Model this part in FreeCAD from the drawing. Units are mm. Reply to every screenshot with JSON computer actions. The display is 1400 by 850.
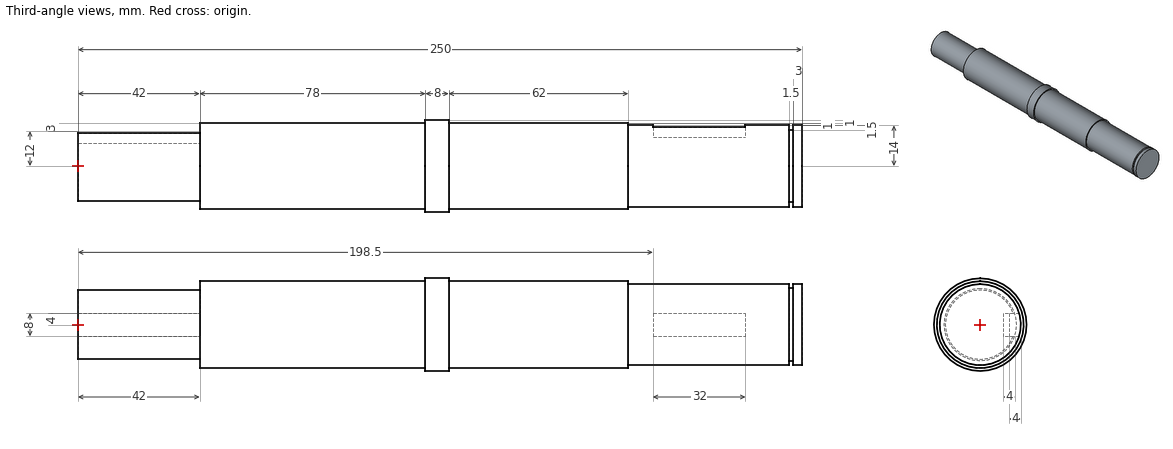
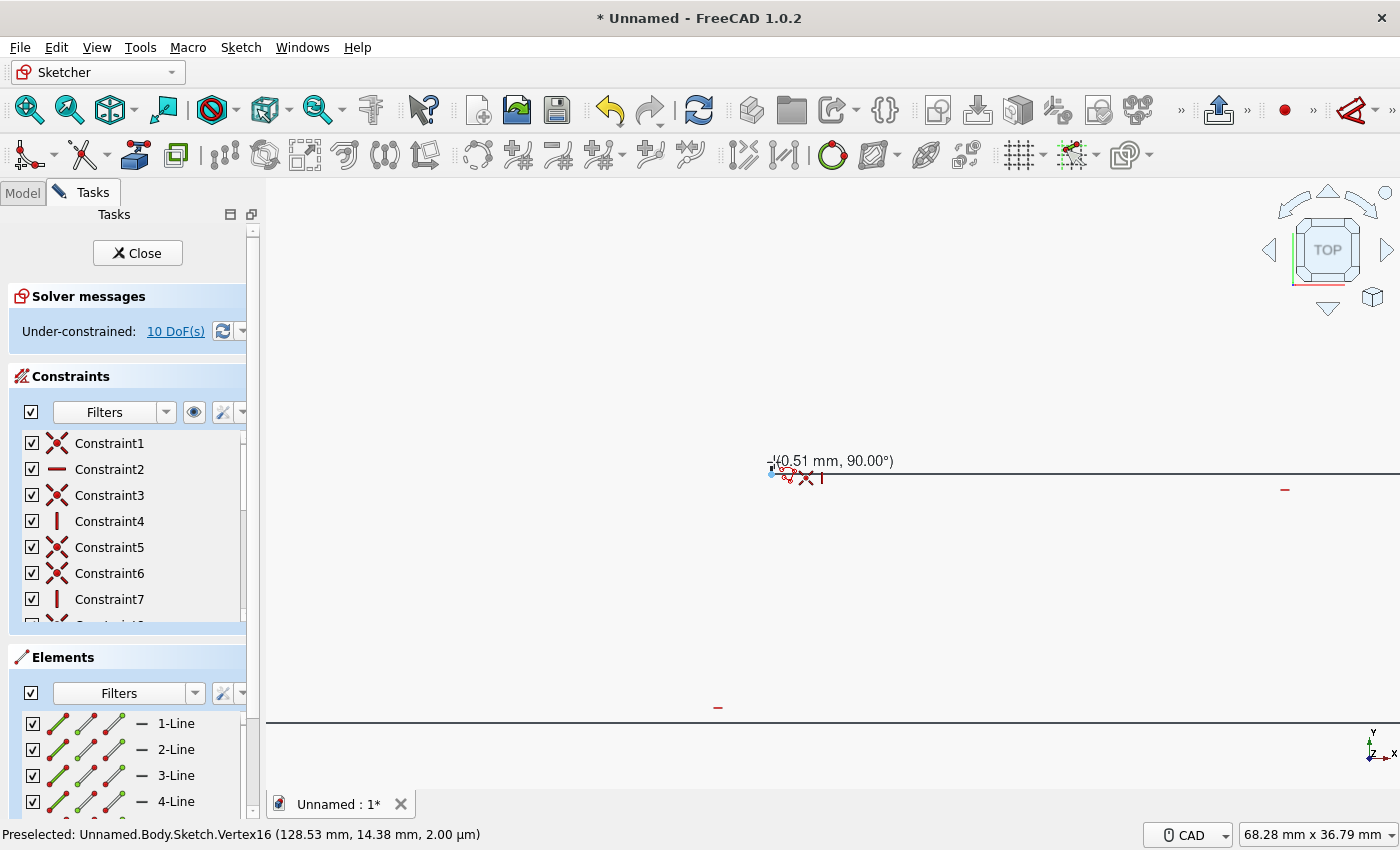
{"action": "left_click", "coordinate": [772, 457]}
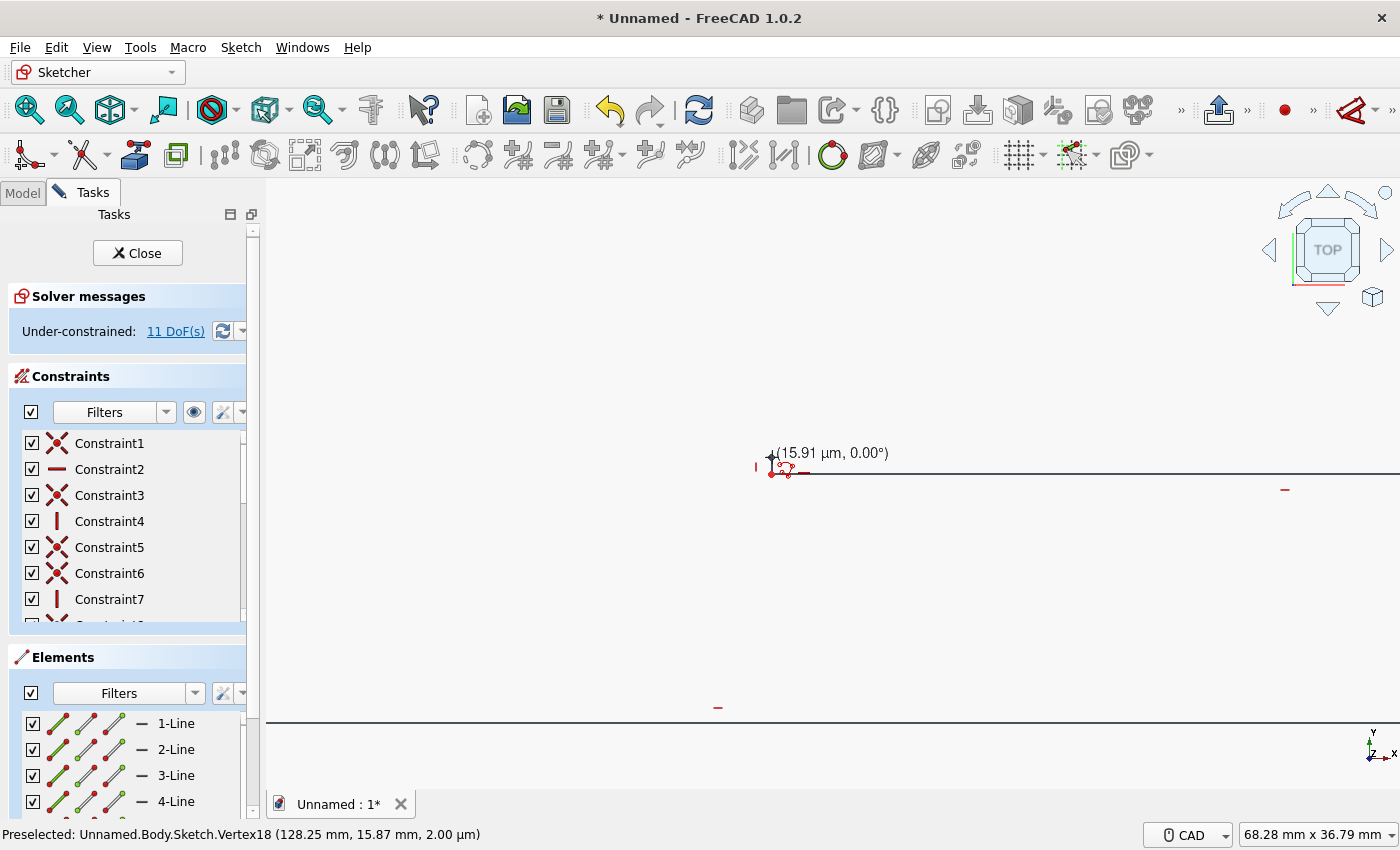
{"action": "scroll", "coordinate": [773, 462], "scroll_direction": "down", "scroll_amount": 9}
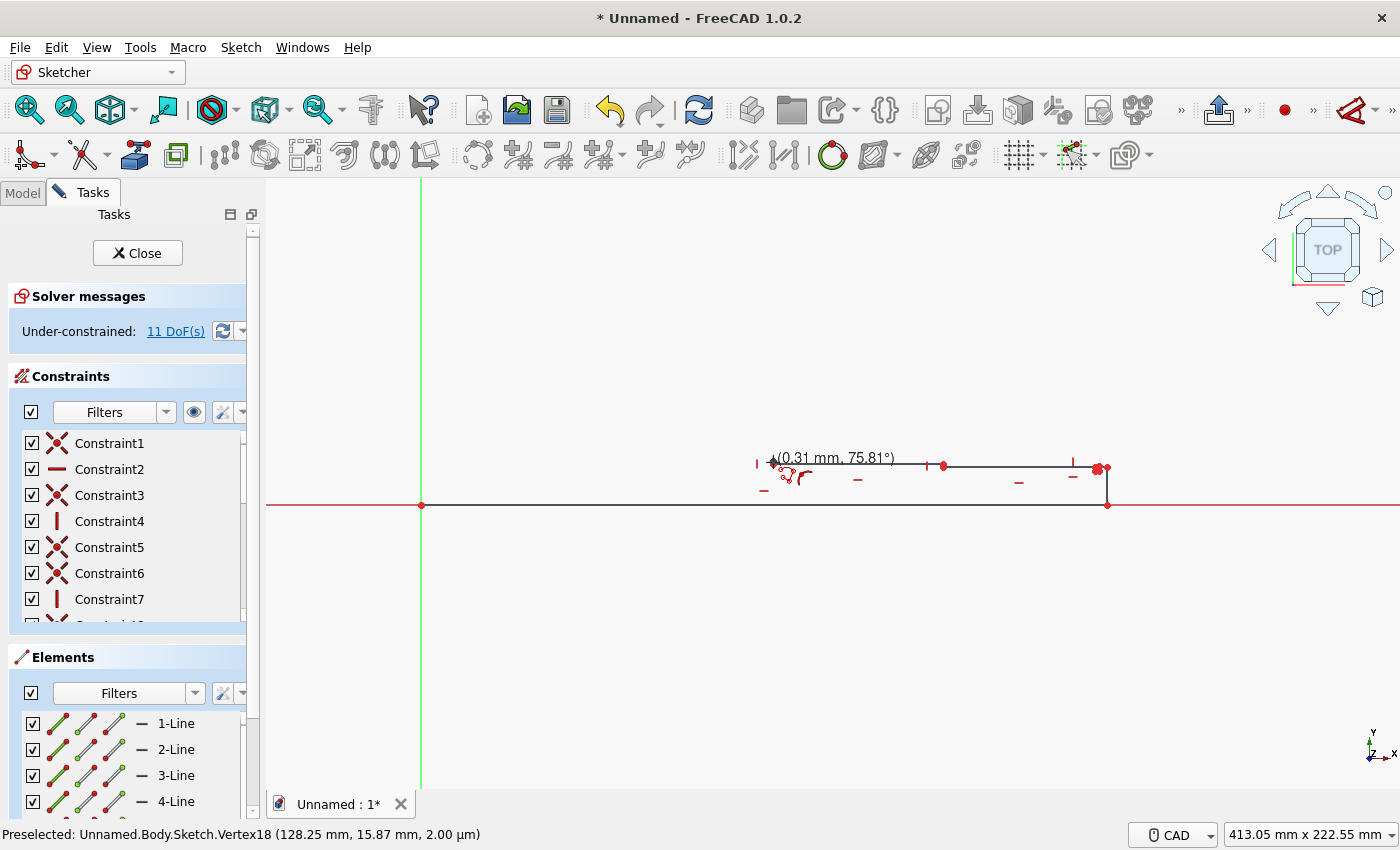
{"action": "left_click", "coordinate": [751, 462]}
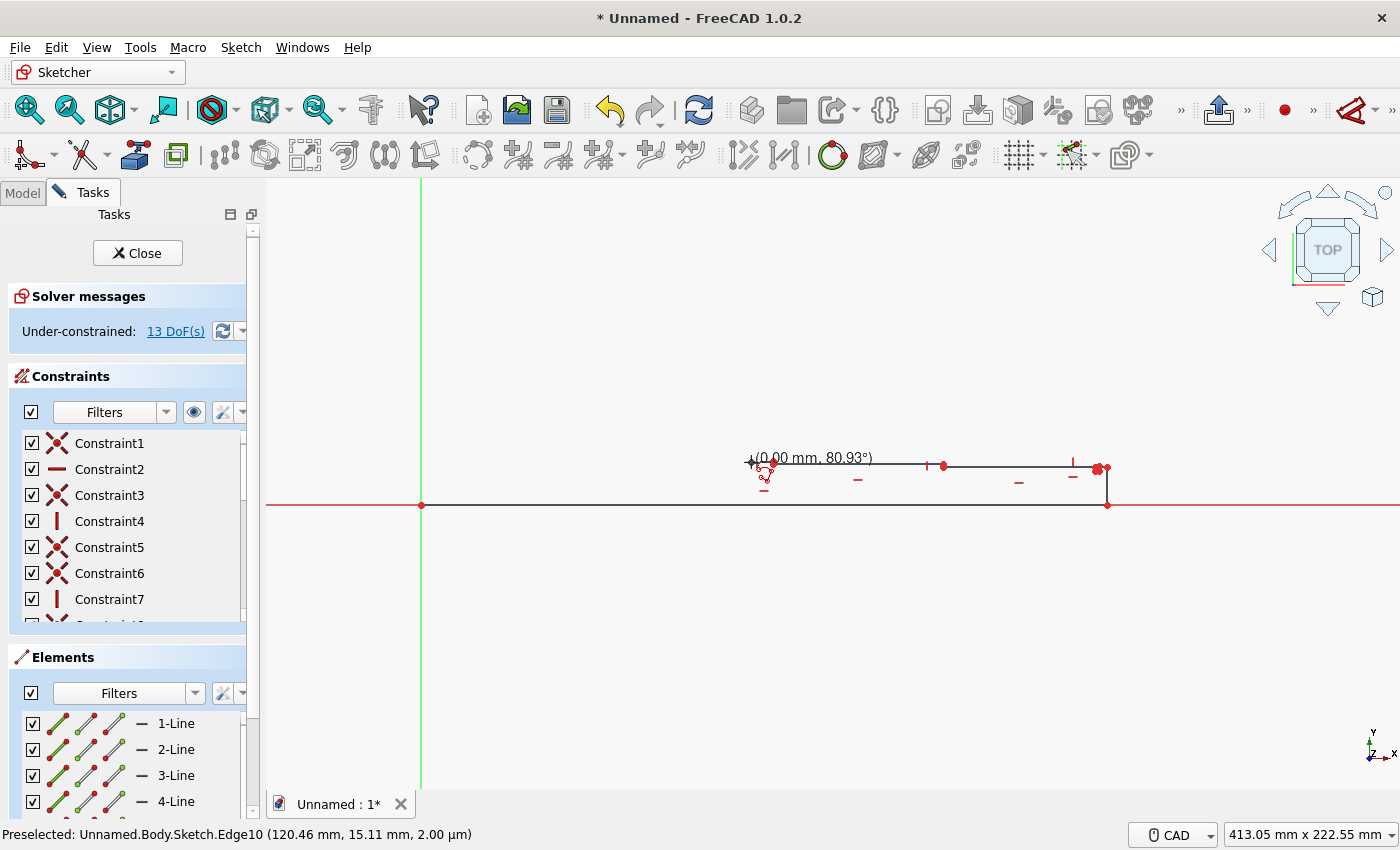
{"action": "scroll", "coordinate": [751, 464], "scroll_direction": "up", "scroll_amount": 9}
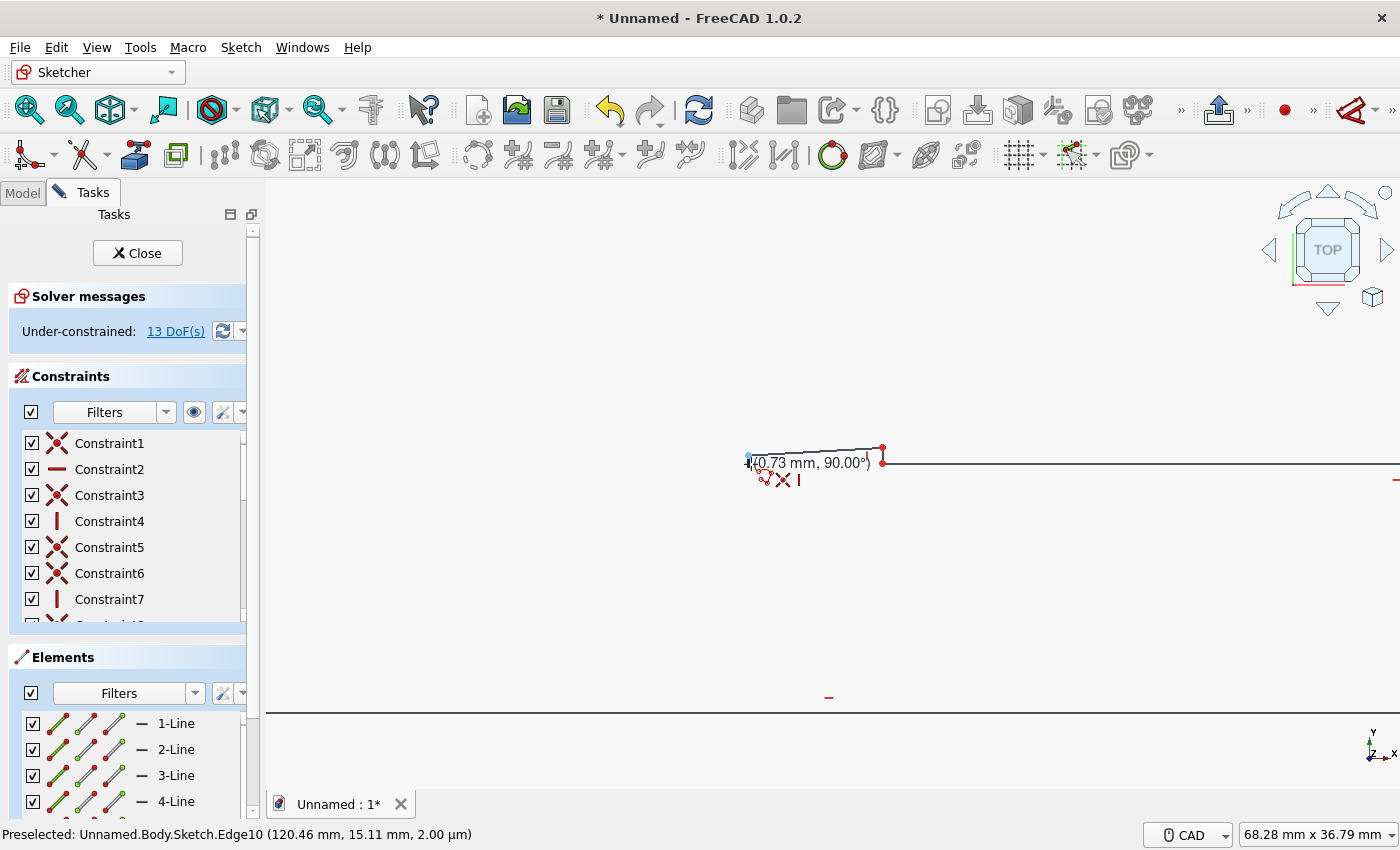
{"action": "left_click", "coordinate": [749, 463]}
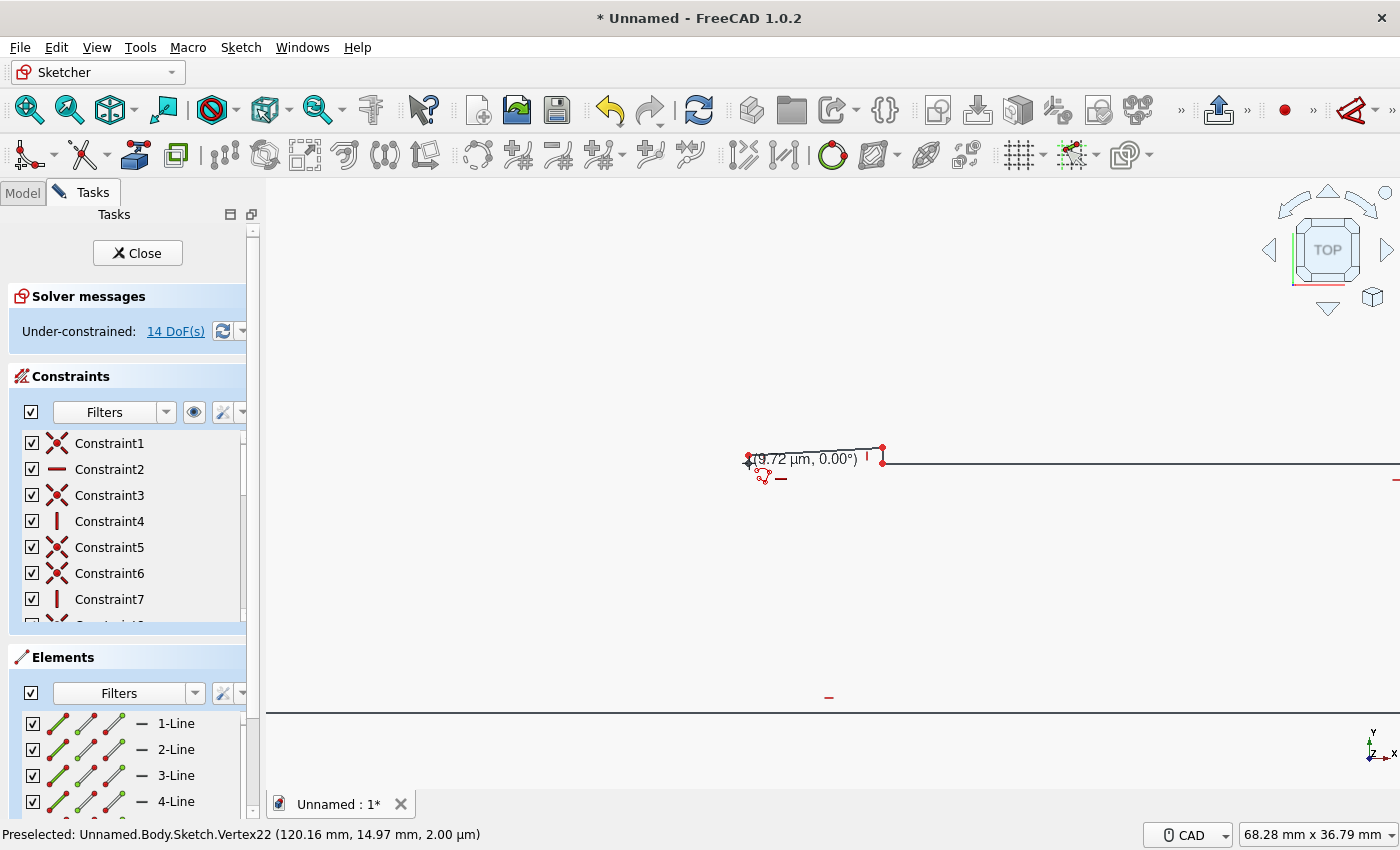
{"action": "scroll", "coordinate": [751, 464], "scroll_direction": "down", "scroll_amount": 9}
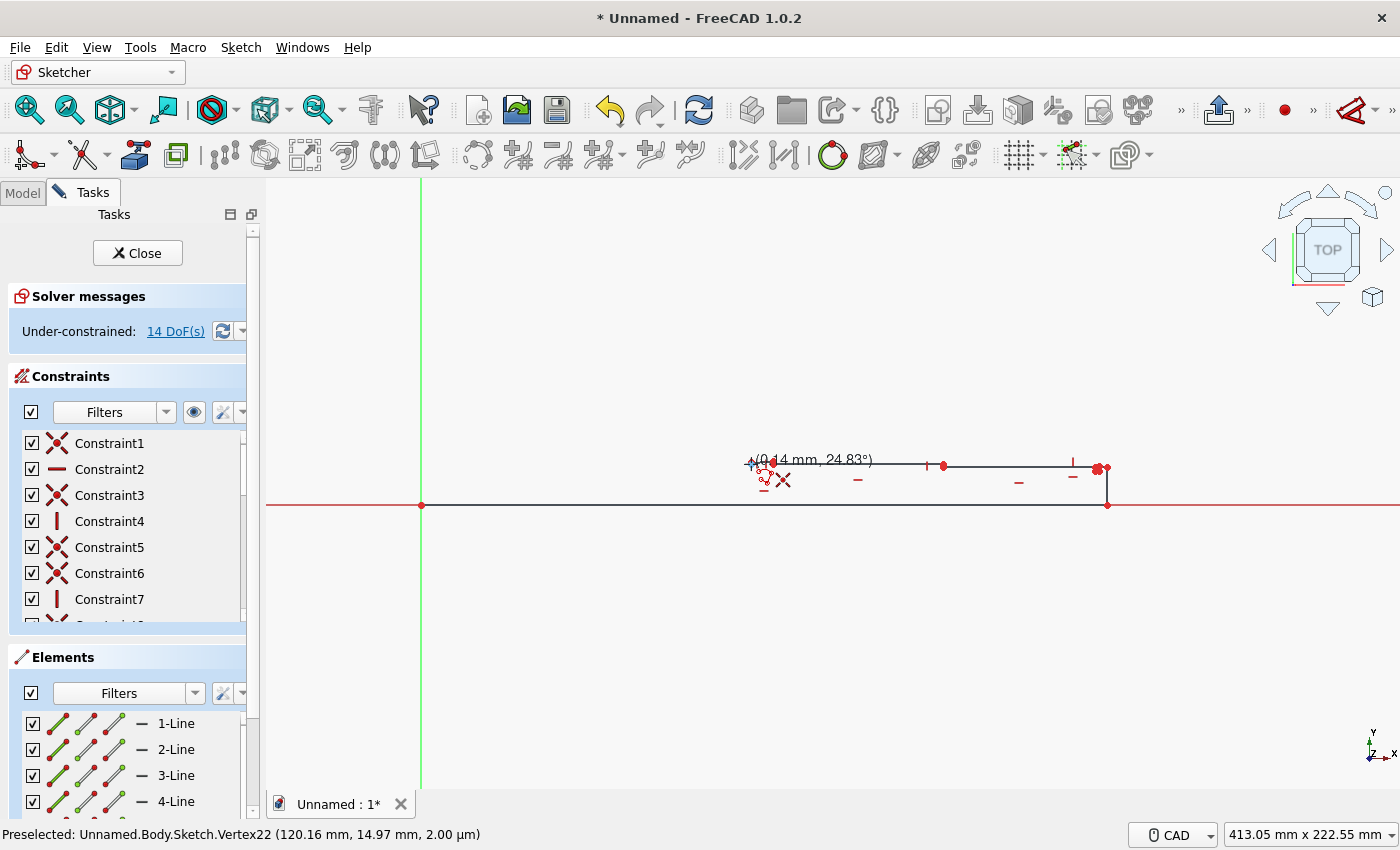
{"action": "left_click", "coordinate": [537, 464]}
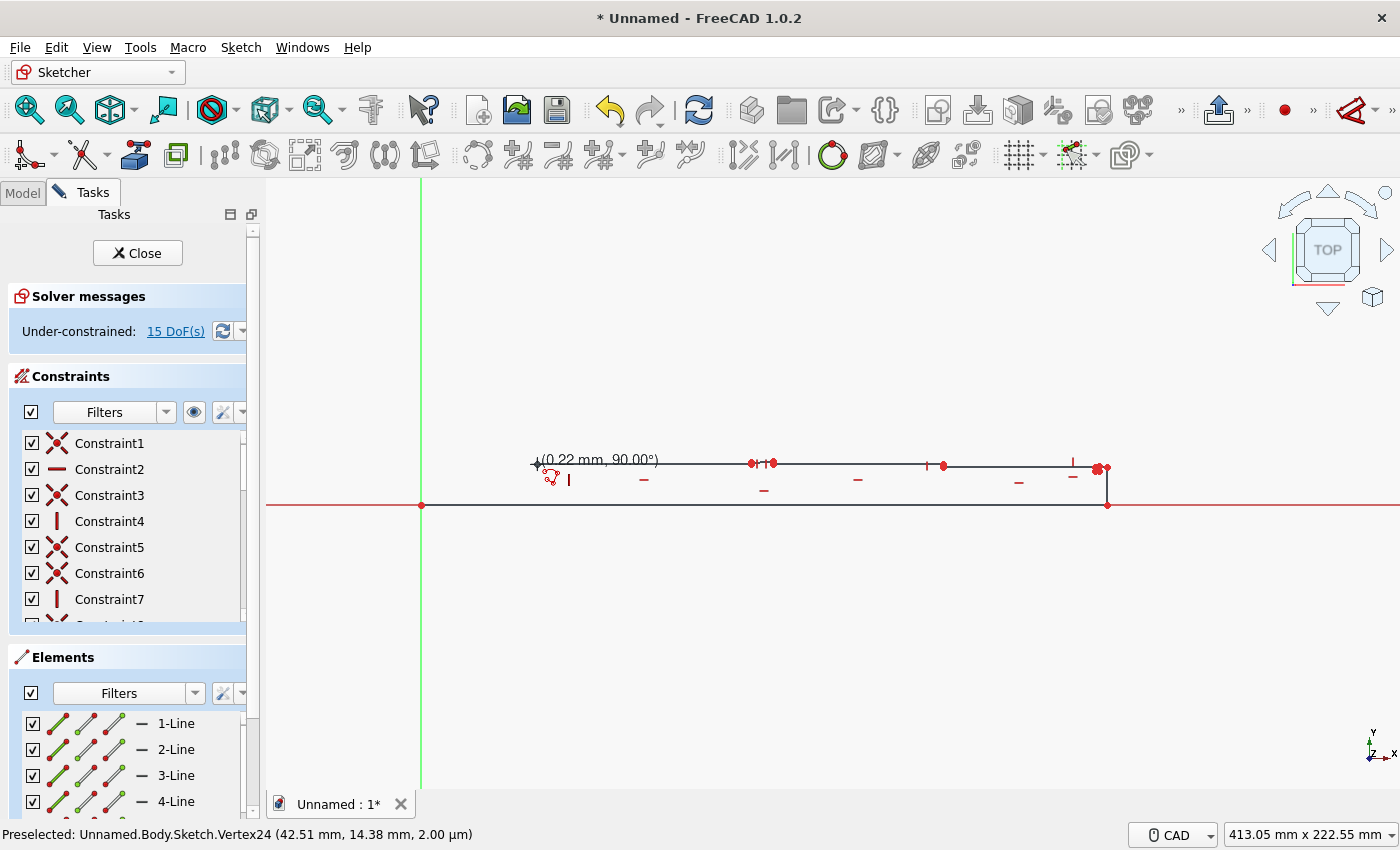
{"action": "scroll", "coordinate": [537, 473], "scroll_direction": "up", "scroll_amount": 4}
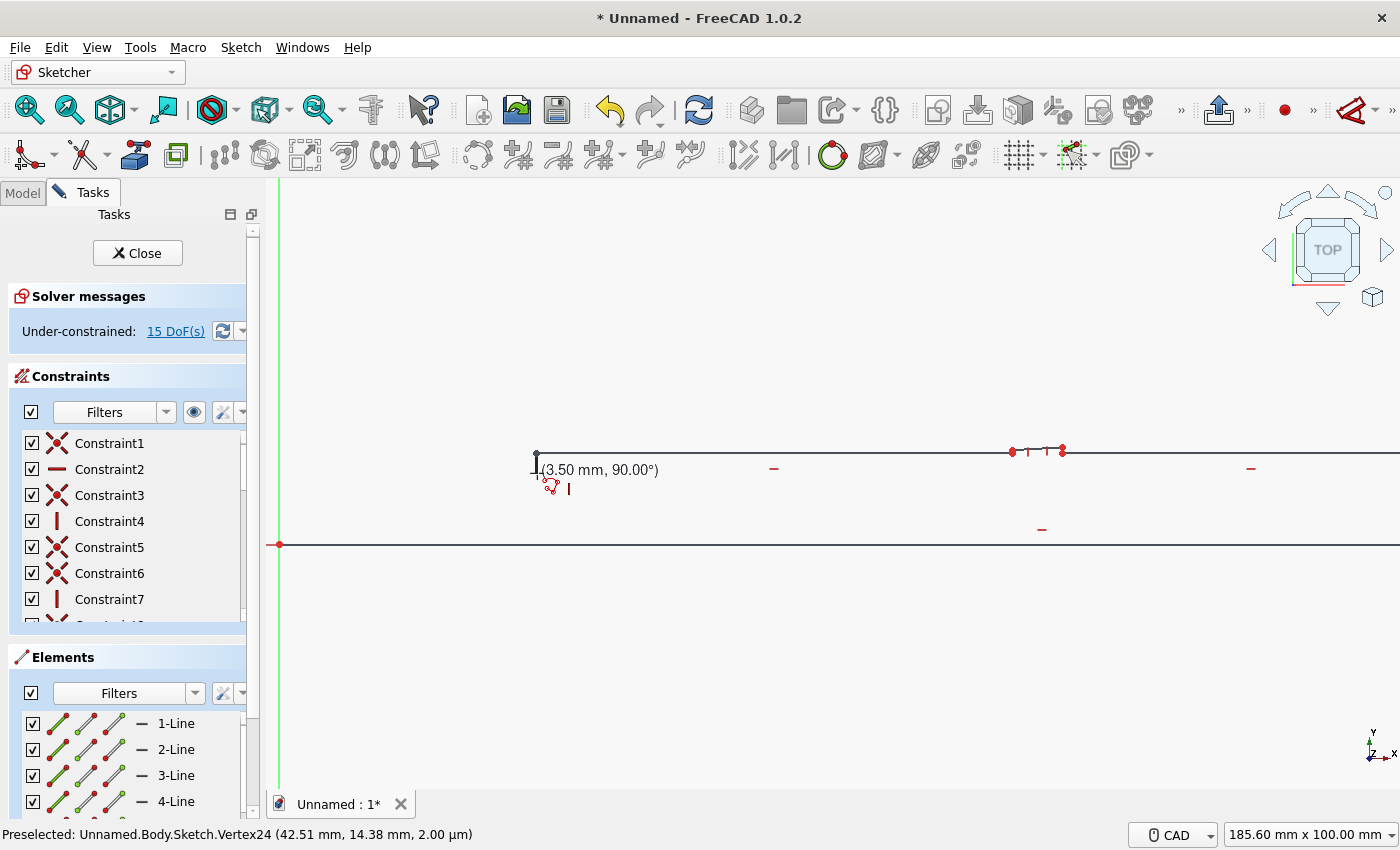
{"action": "left_click", "coordinate": [537, 471]}